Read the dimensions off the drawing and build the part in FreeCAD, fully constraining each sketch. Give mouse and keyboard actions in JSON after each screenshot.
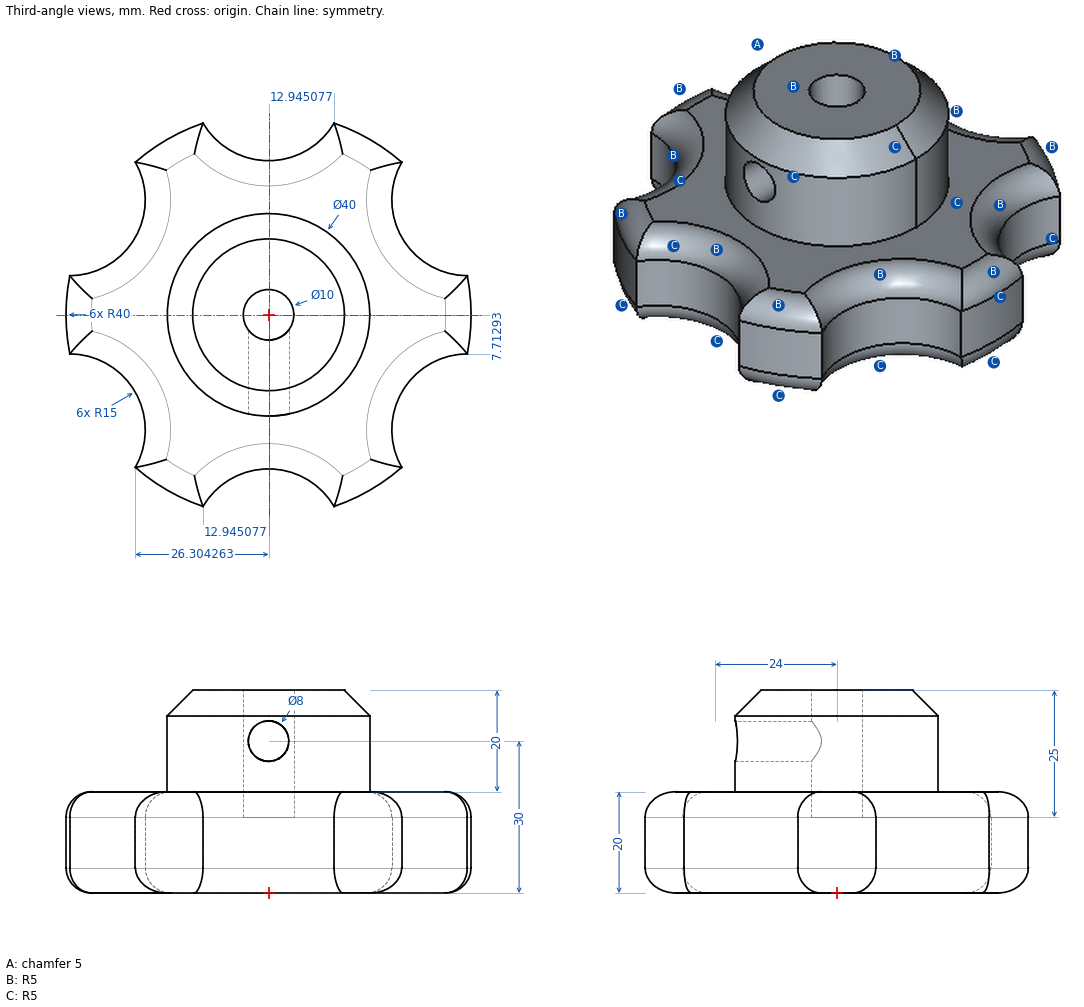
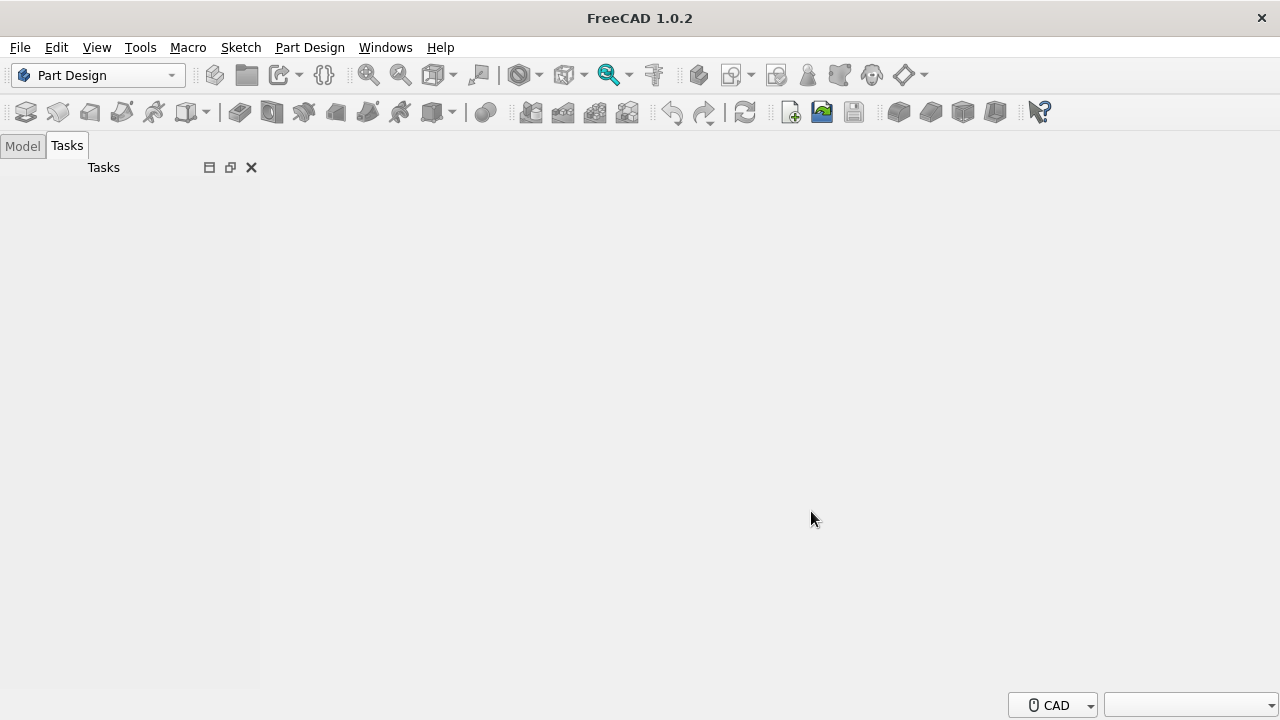
{"action": "left_click", "coordinate": [790, 112]}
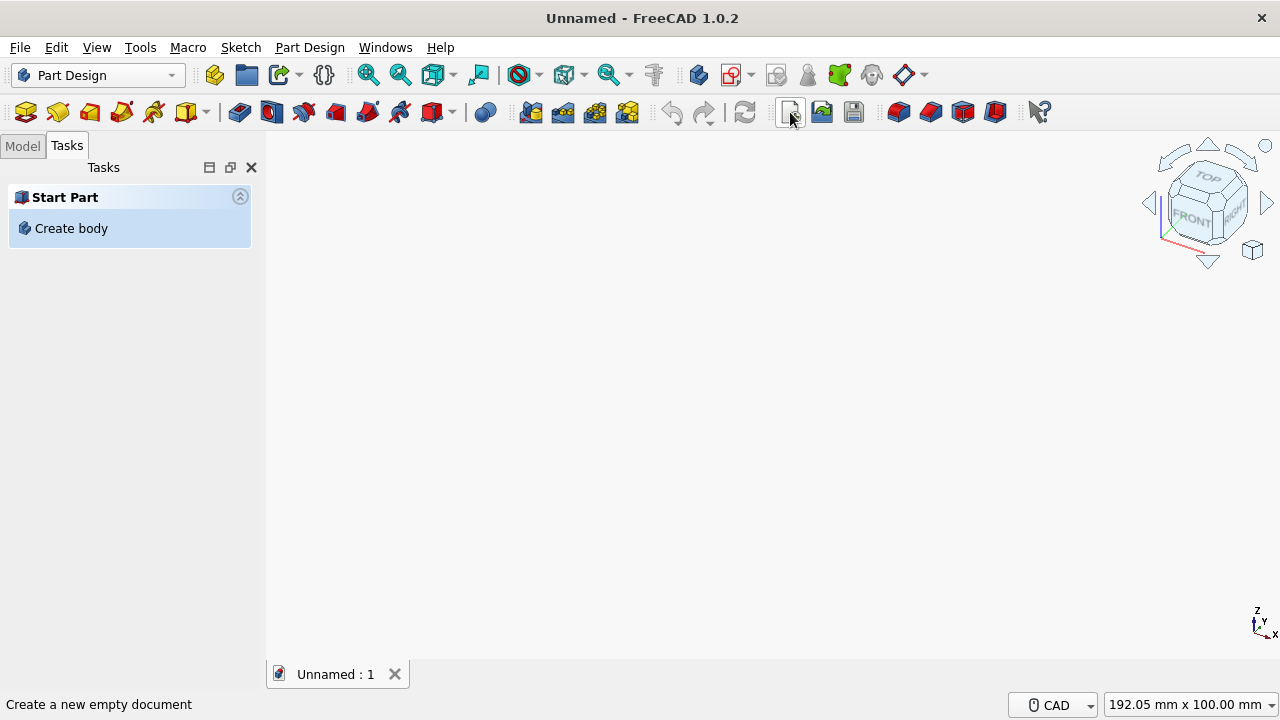
{"action": "left_click", "coordinate": [732, 76]}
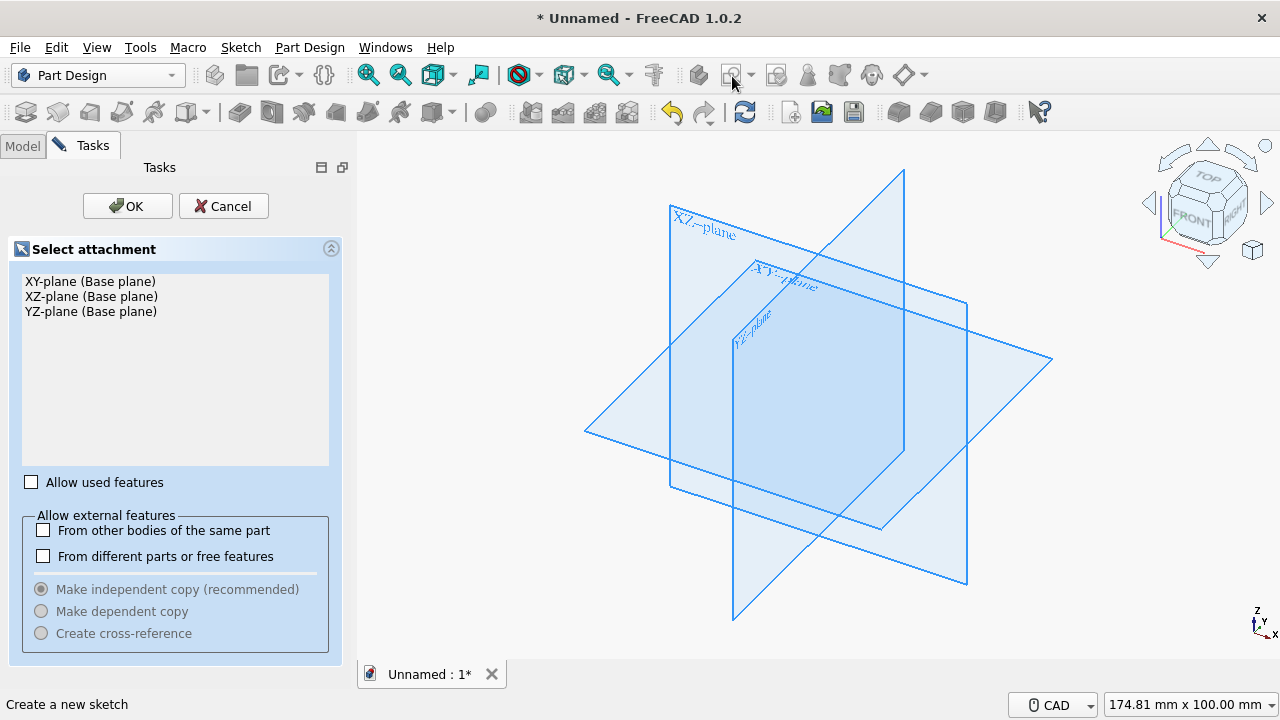
{"action": "left_click", "coordinate": [82, 282]}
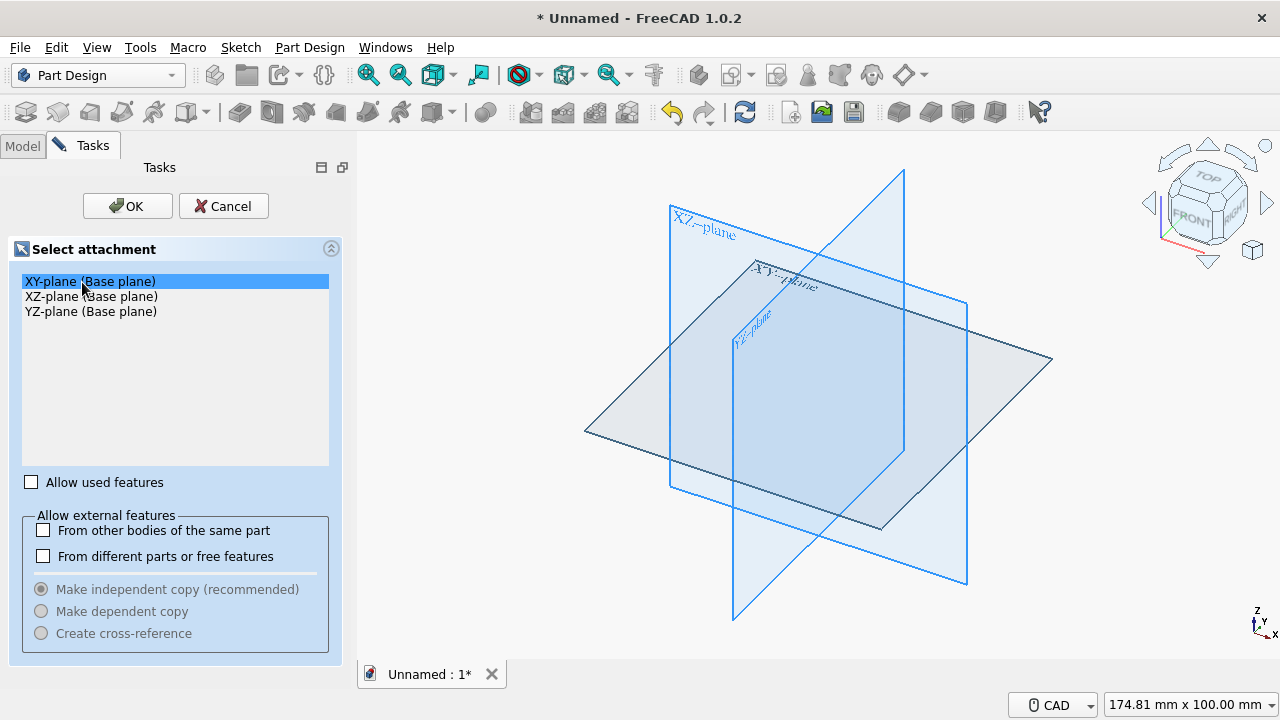
{"action": "left_click", "coordinate": [128, 206]}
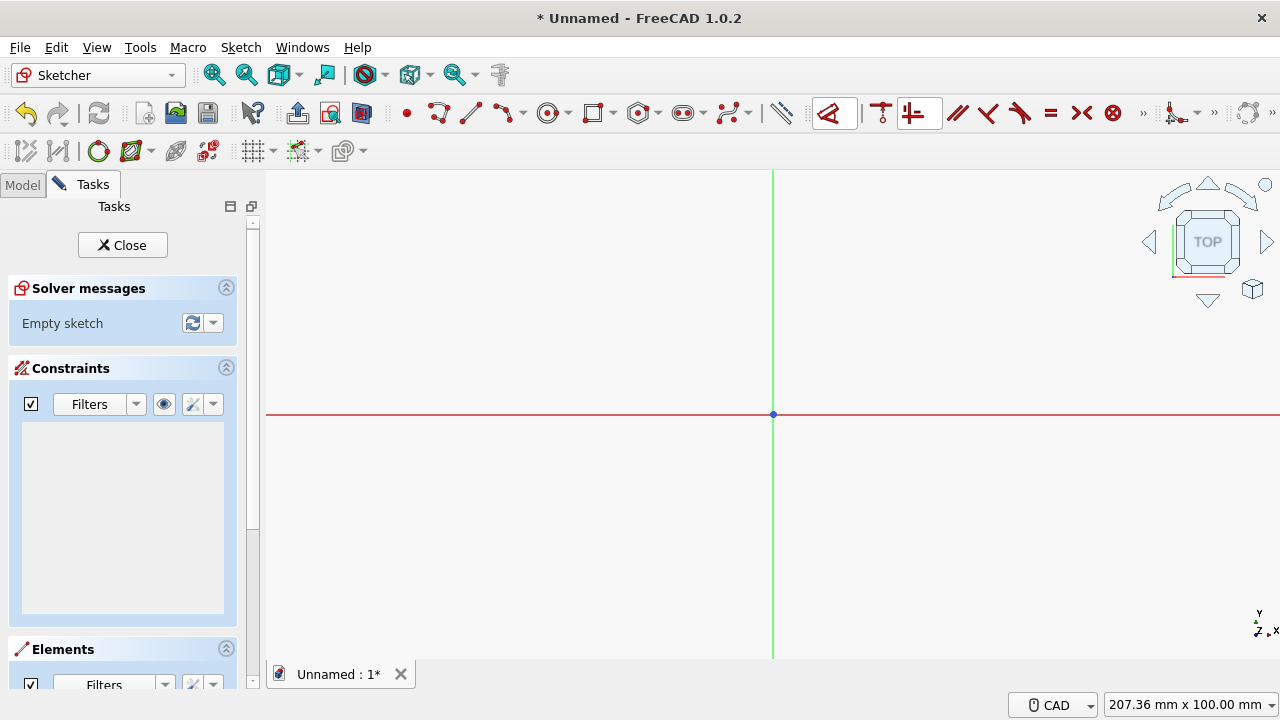
{"action": "left_click", "coordinate": [504, 114]}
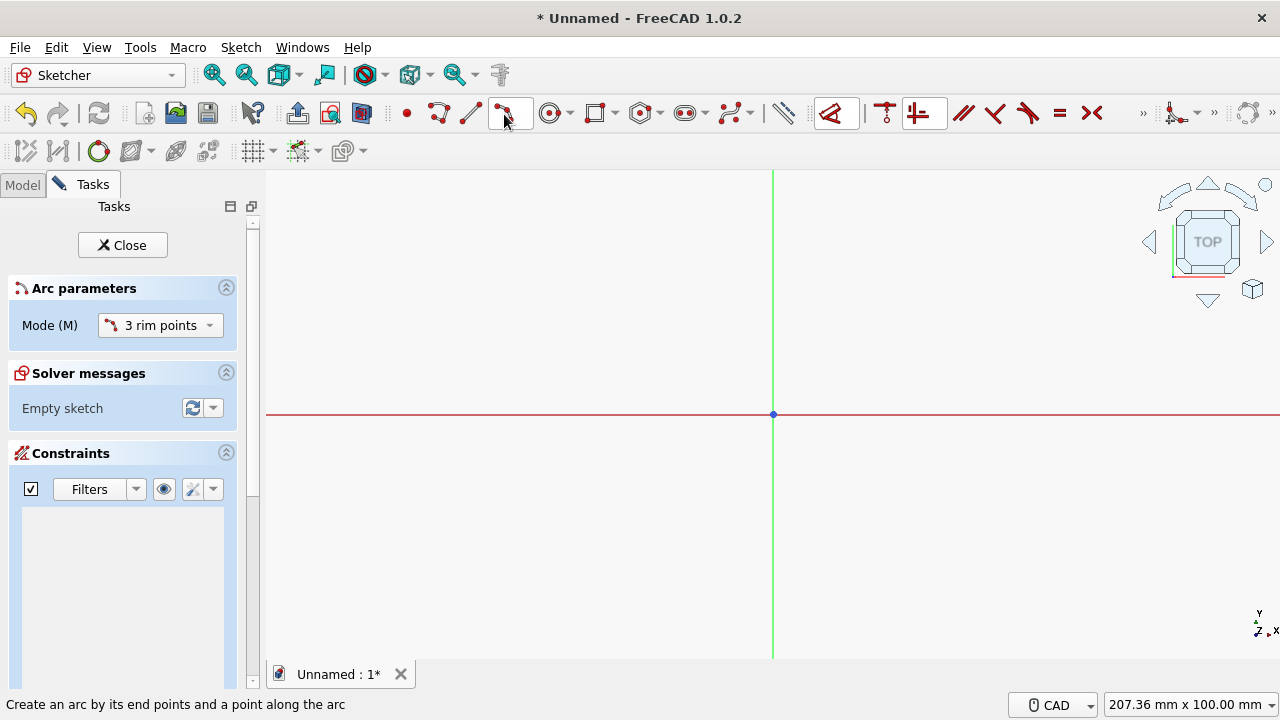
{"action": "left_click", "coordinate": [644, 562]}
{"action": "left_click", "coordinate": [710, 600]}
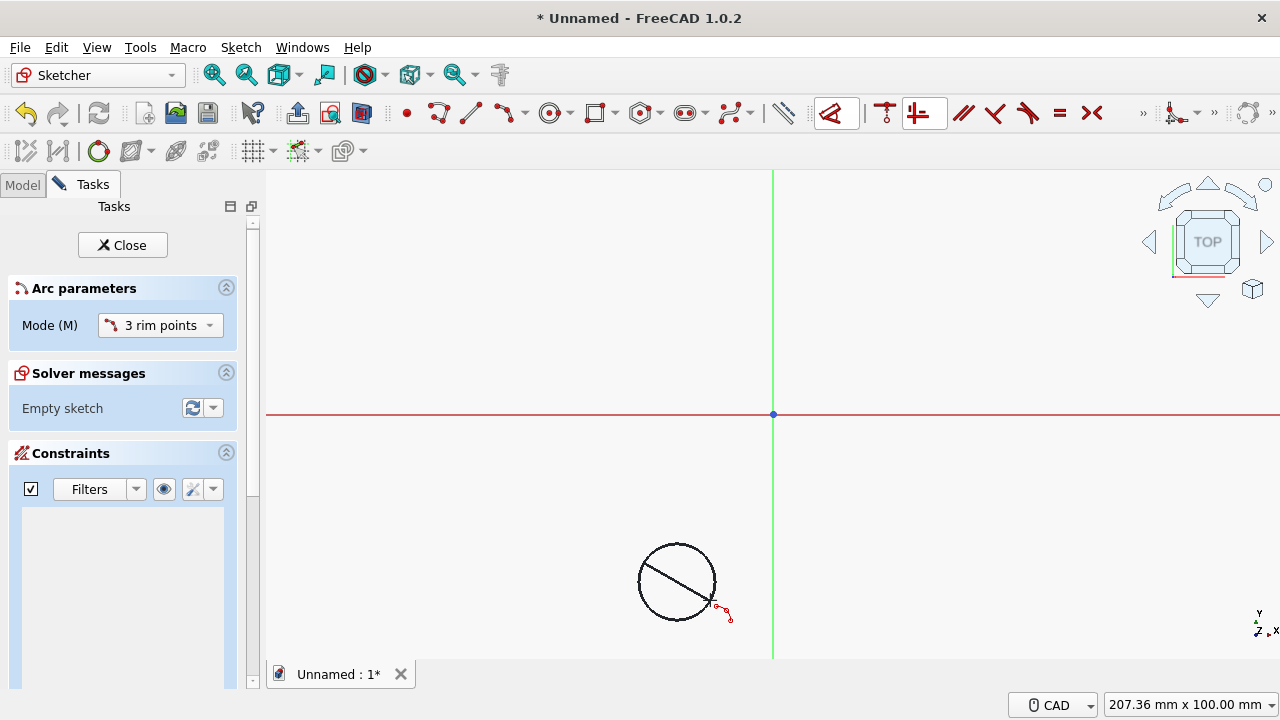
{"action": "scroll", "coordinate": [675, 584], "scroll_direction": "up", "scroll_amount": 8}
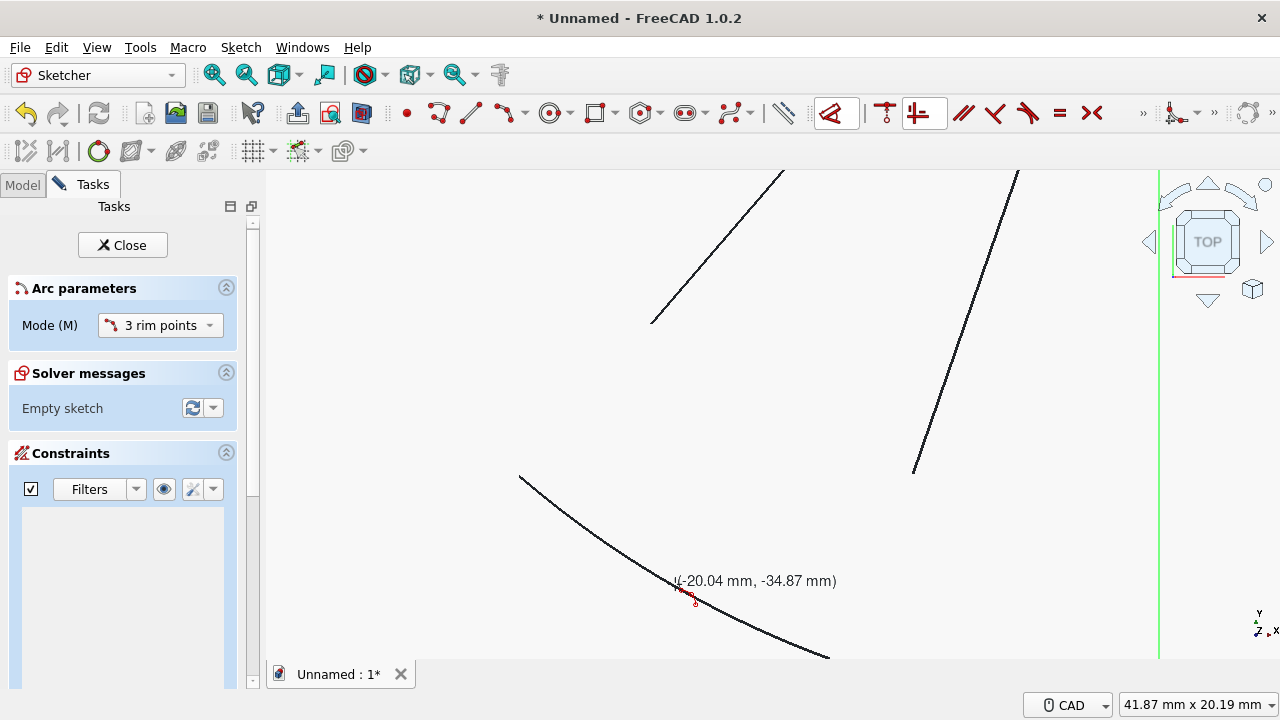
{"action": "left_click", "coordinate": [674, 580]}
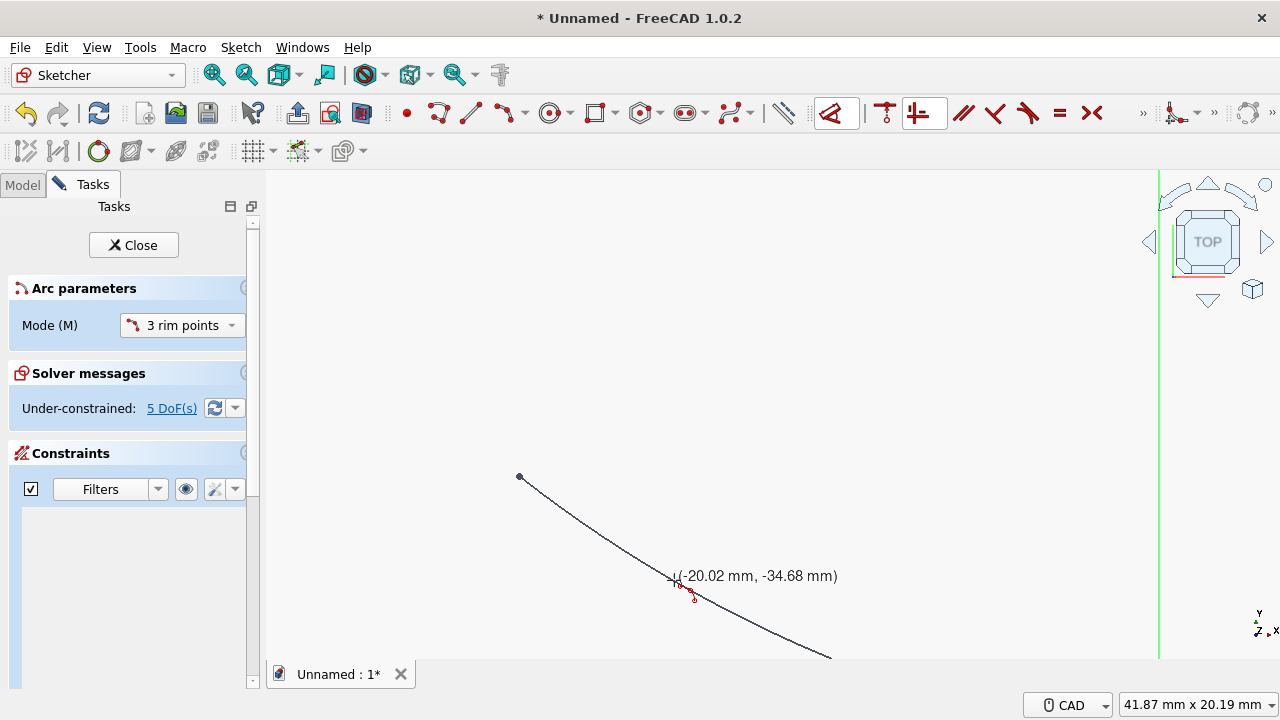
{"action": "scroll", "coordinate": [615, 548], "scroll_direction": "down", "scroll_amount": 9}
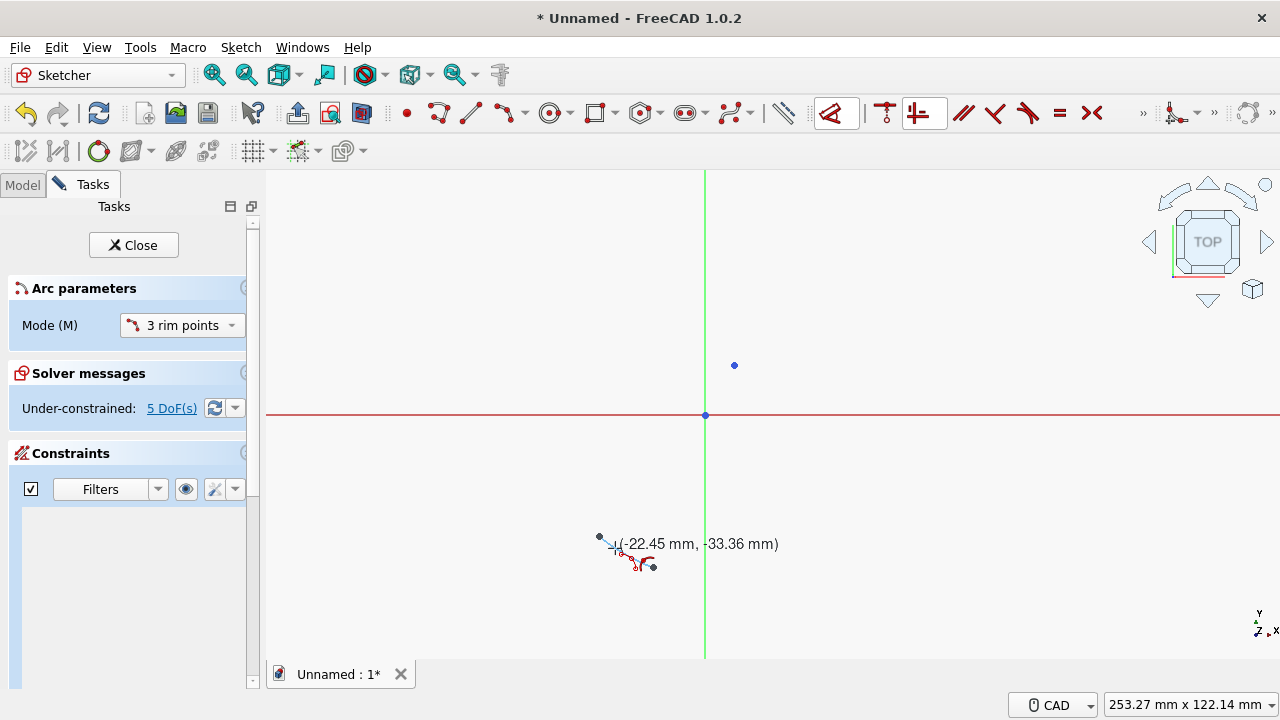
{"action": "left_click", "coordinate": [654, 568]}
{"action": "left_click", "coordinate": [757, 567]}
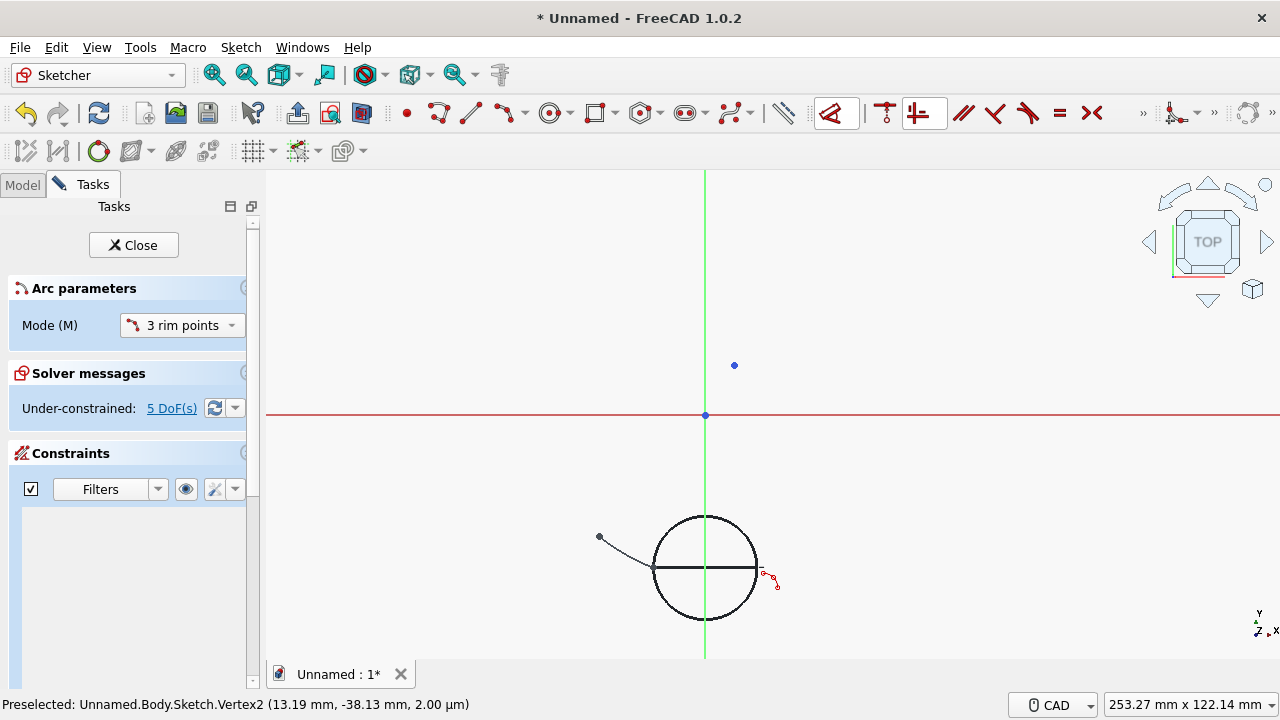
{"action": "scroll", "coordinate": [718, 538], "scroll_direction": "up", "scroll_amount": 2}